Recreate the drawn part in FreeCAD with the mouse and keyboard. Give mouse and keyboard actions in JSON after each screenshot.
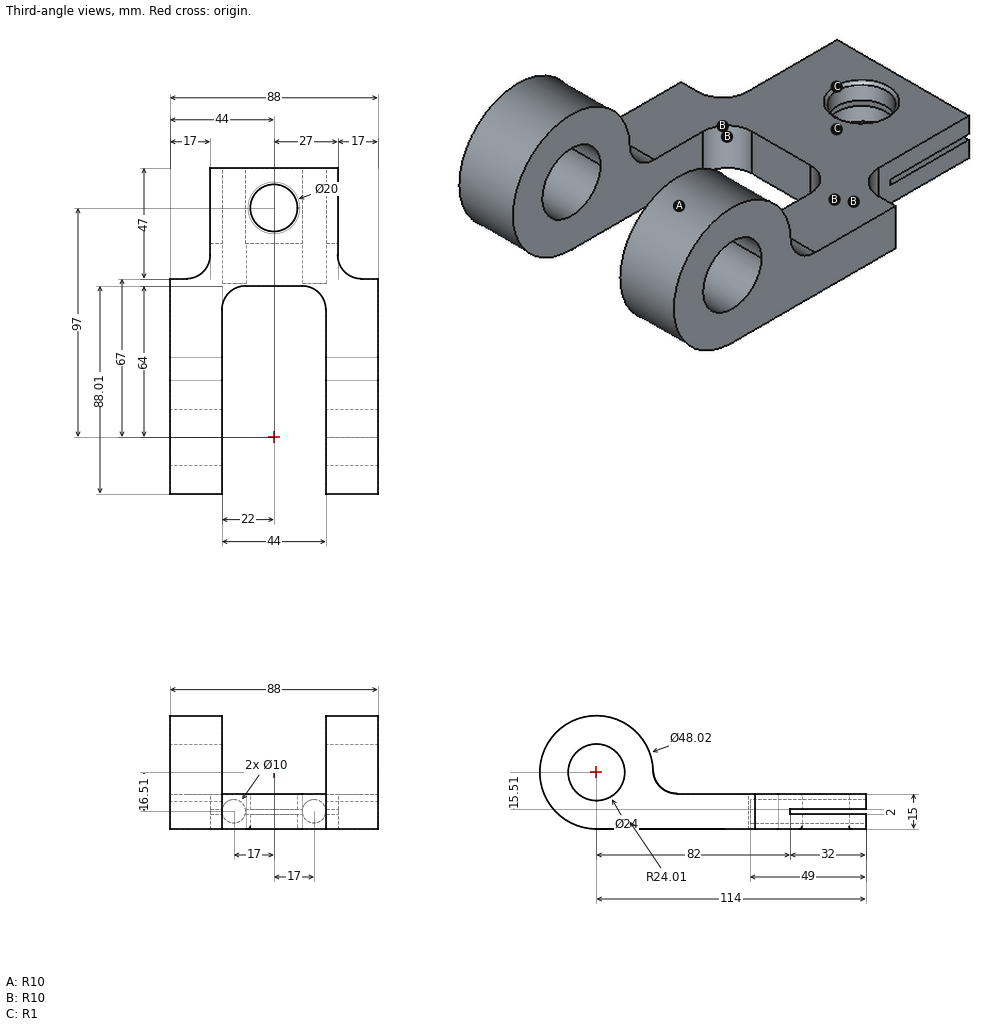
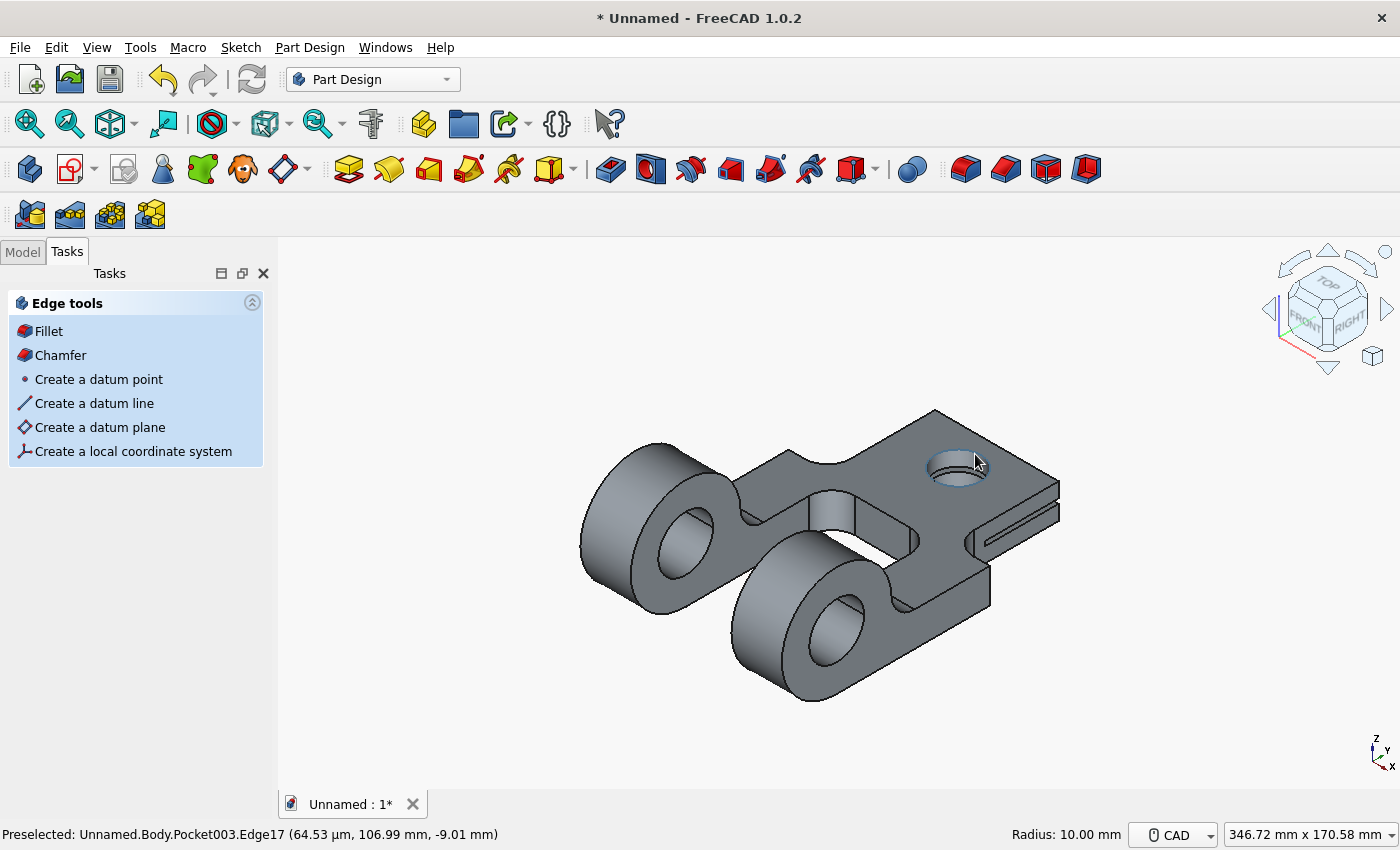
{"action": "key", "text": "1"}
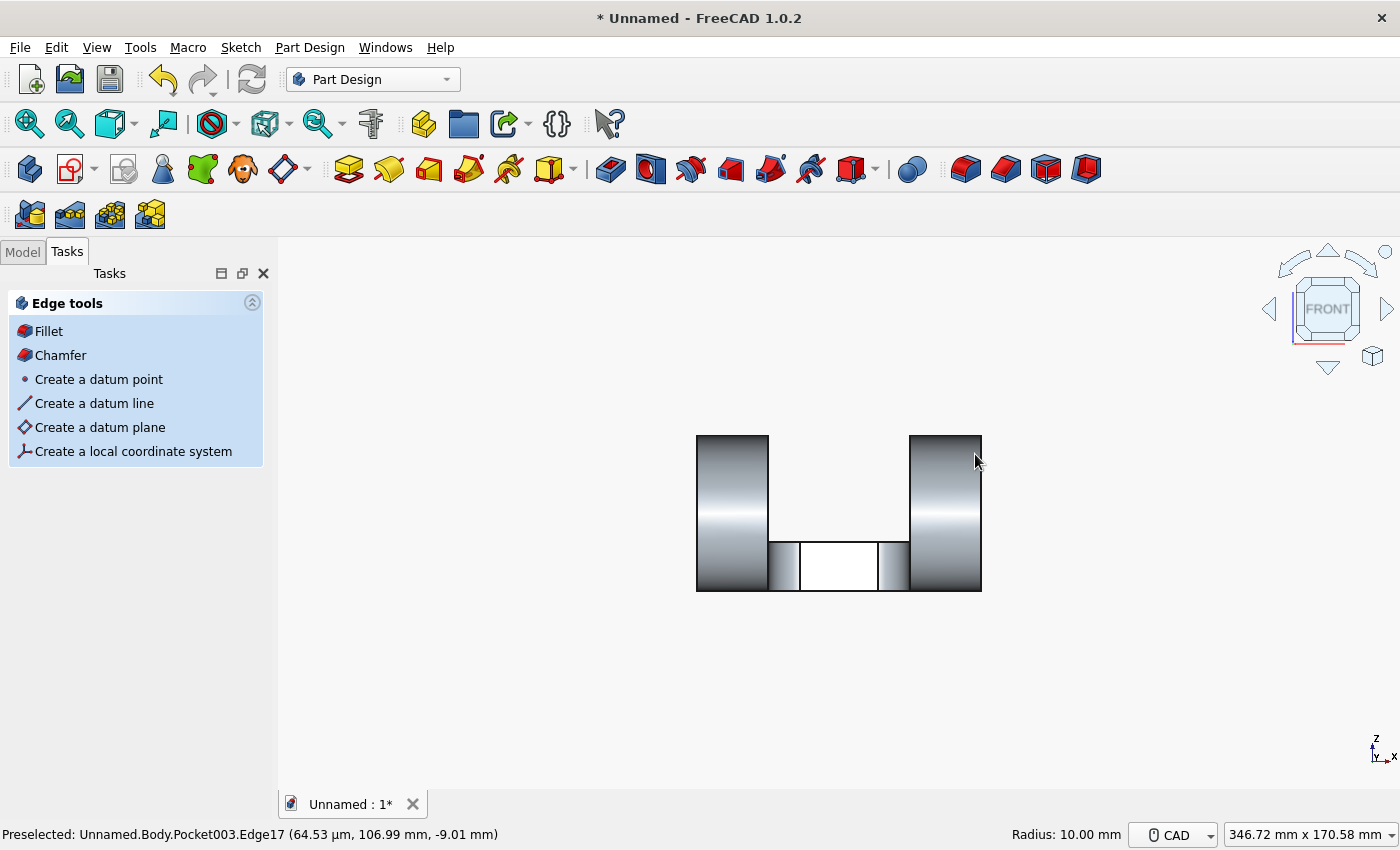
{"action": "left_click", "coordinate": [30, 124]}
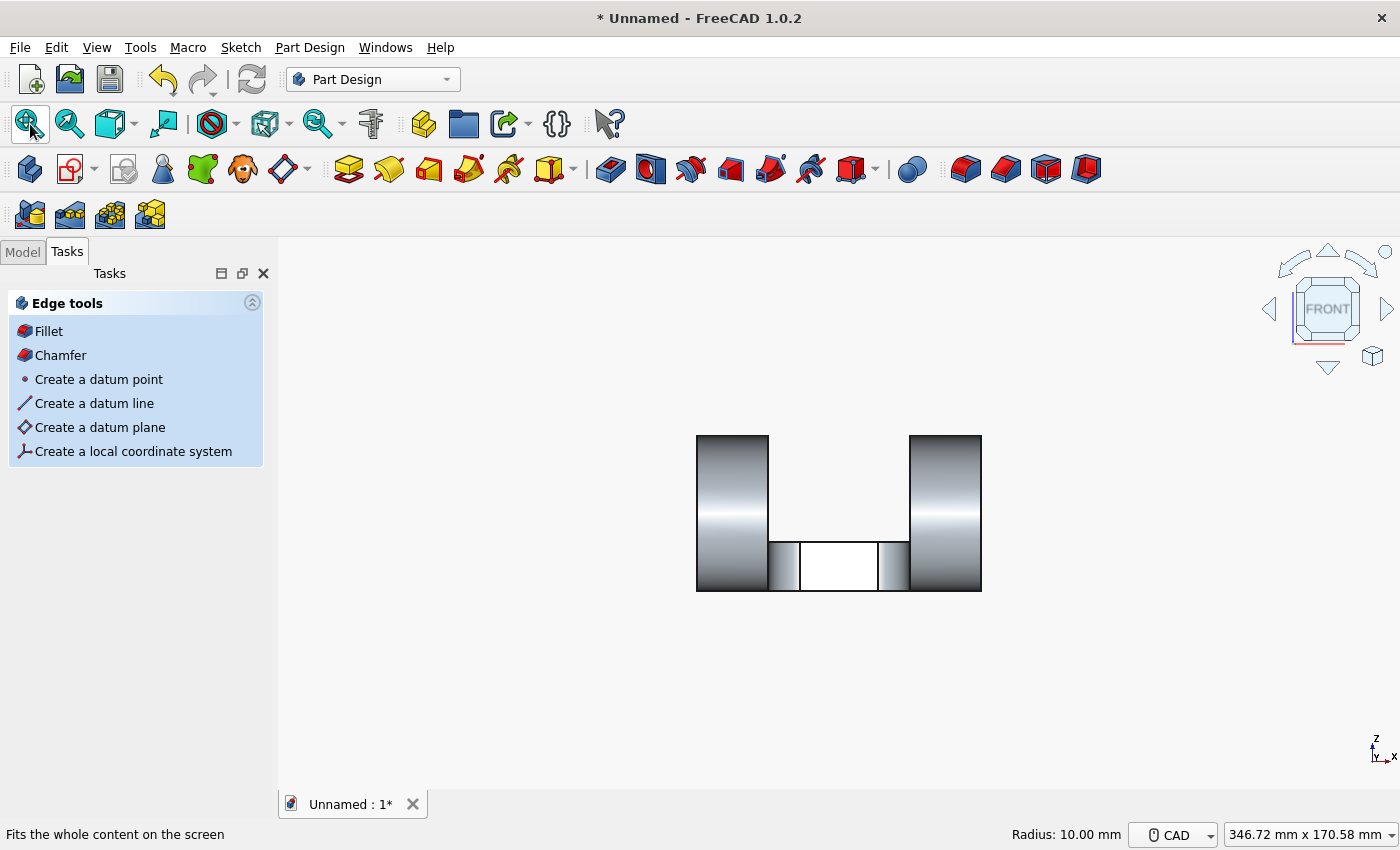
{"action": "key", "text": "3"}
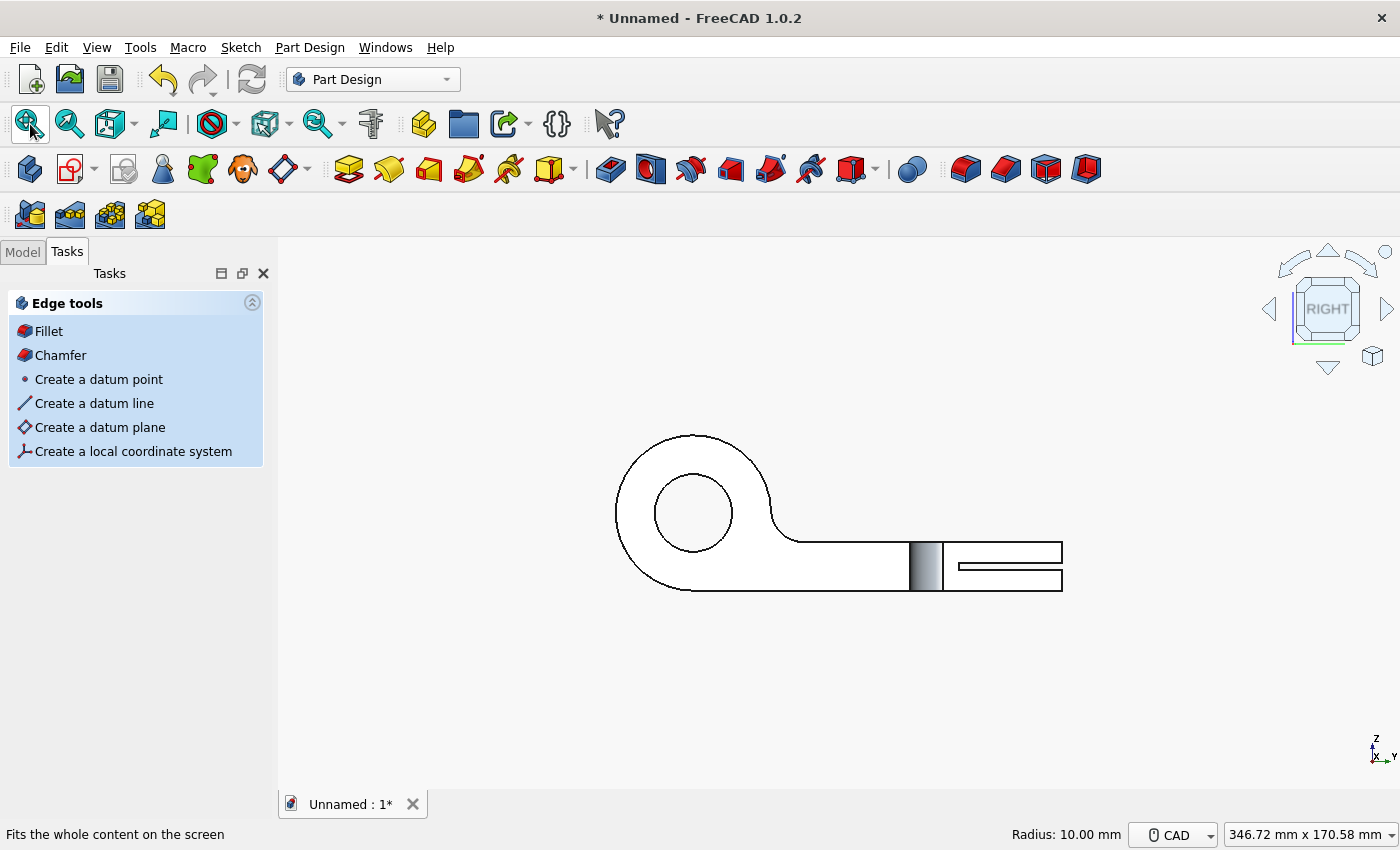
{"action": "left_click", "coordinate": [30, 124]}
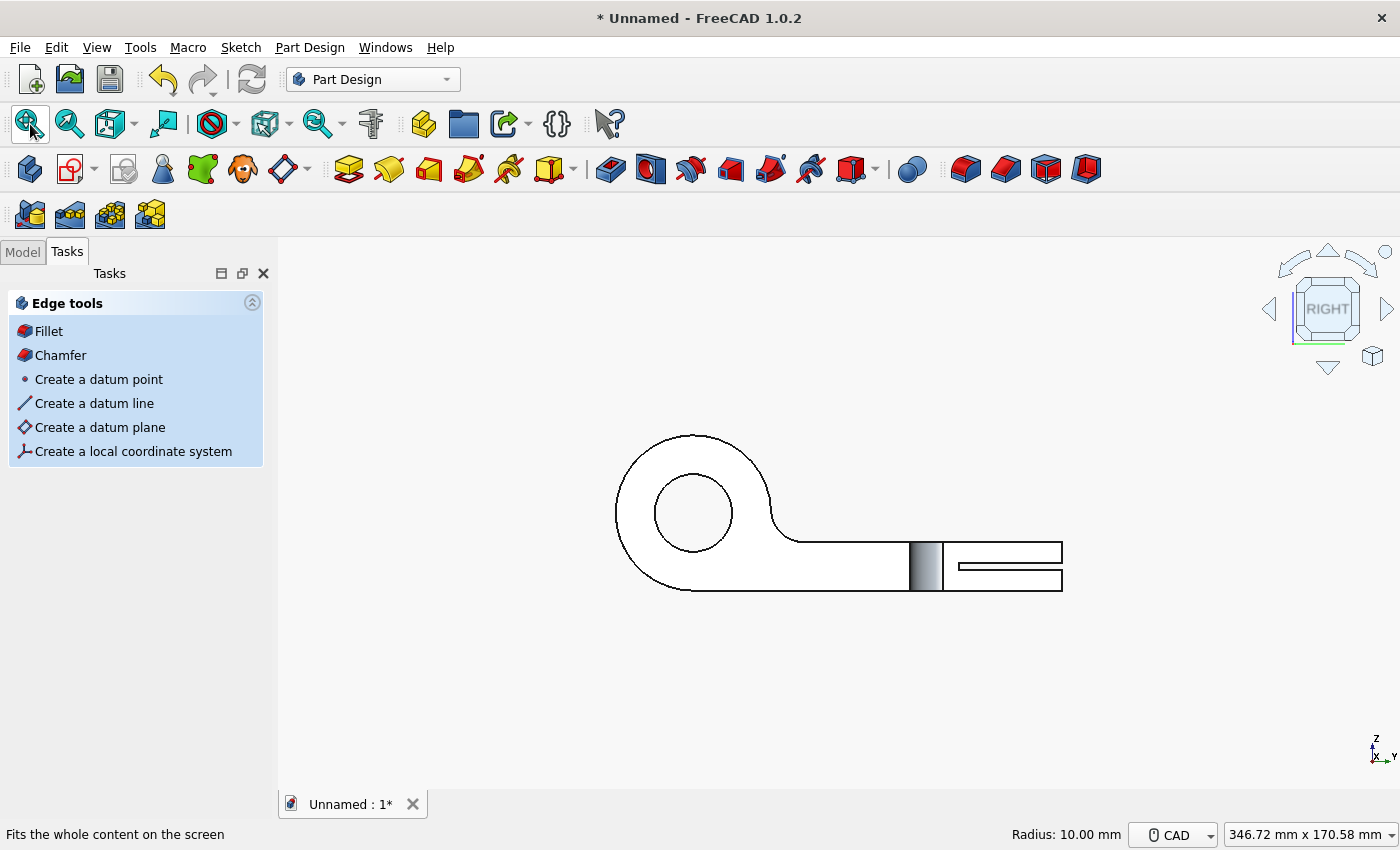
{"action": "key", "text": "5"}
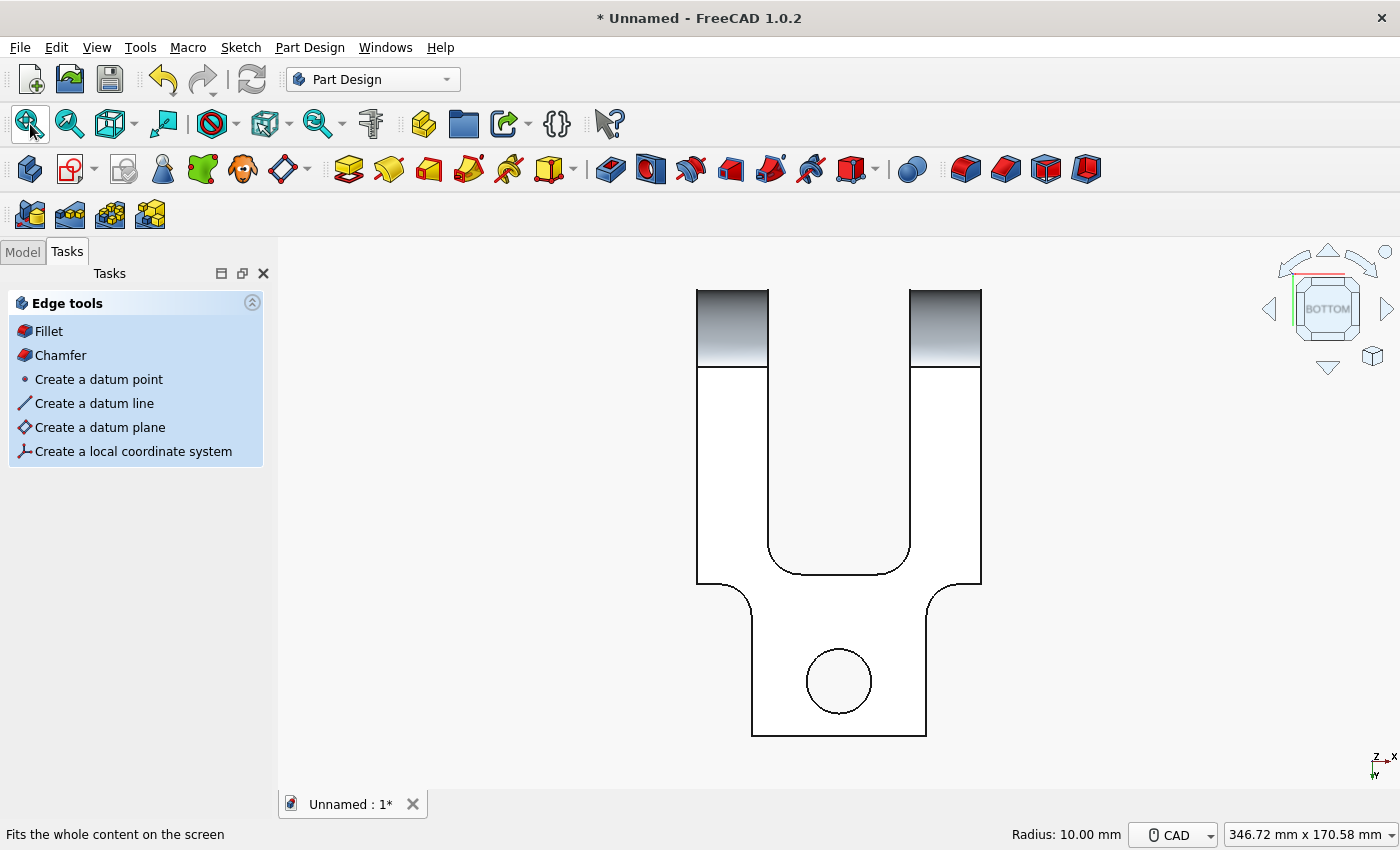
{"action": "left_click", "coordinate": [839, 713], "text": "ctrl"}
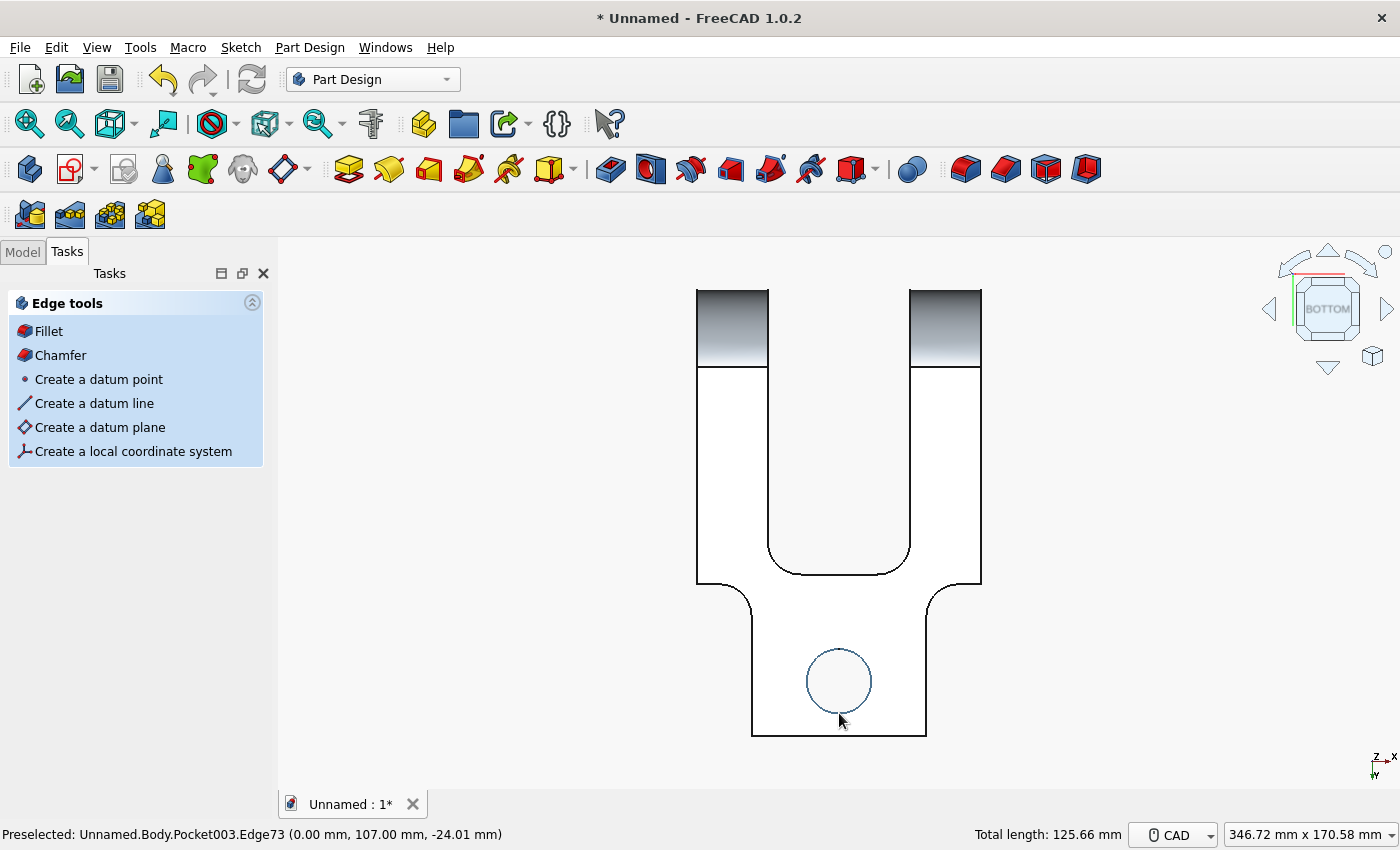
{"action": "left_click", "coordinate": [966, 170]}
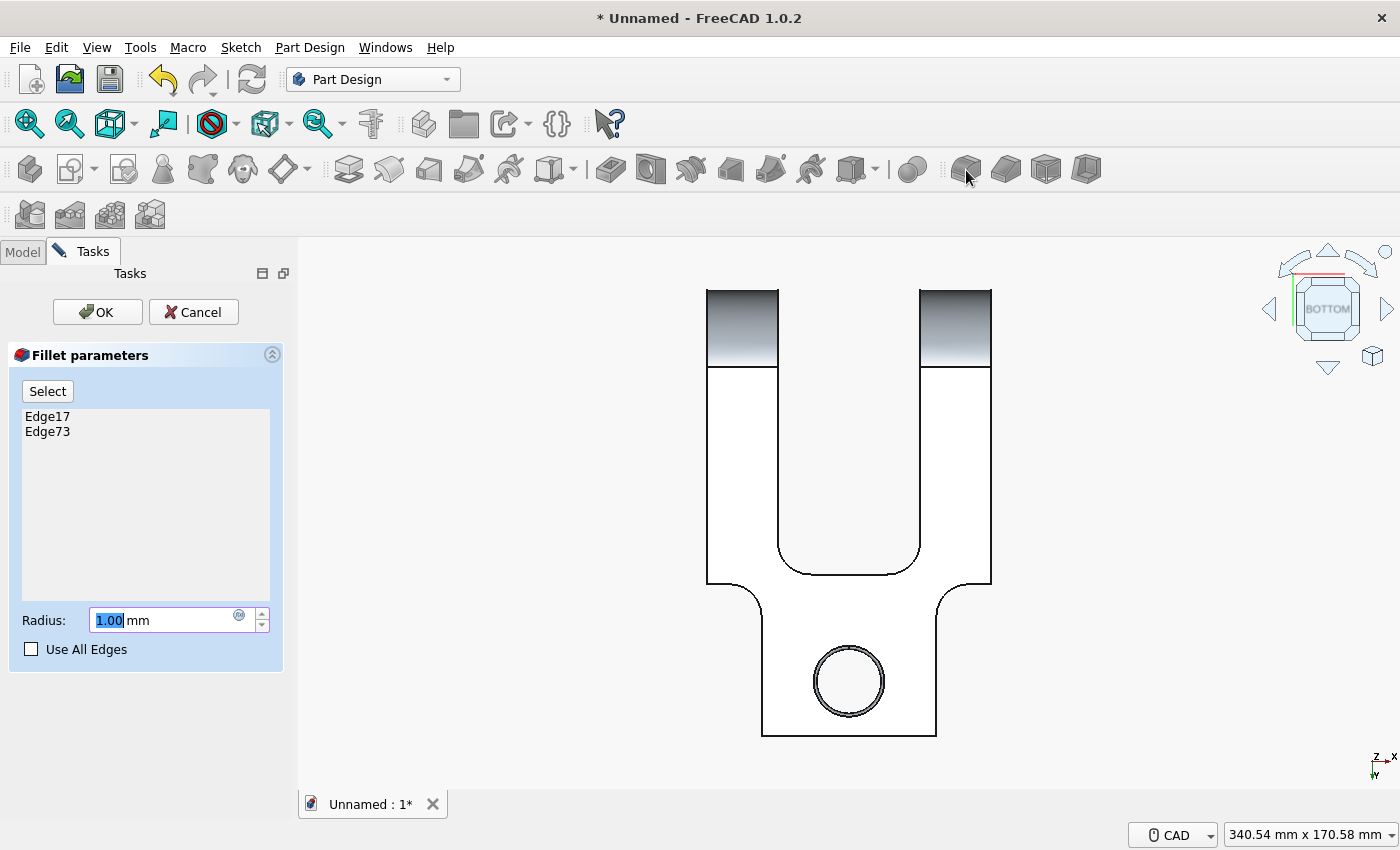
{"action": "type", "text": "1"}
{"action": "key", "text": "Tab"}